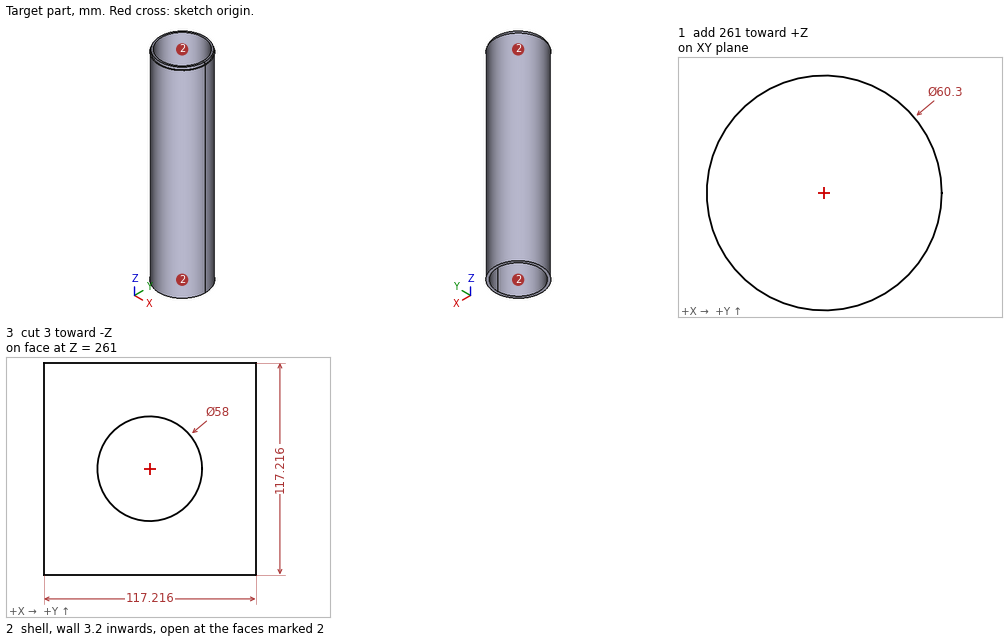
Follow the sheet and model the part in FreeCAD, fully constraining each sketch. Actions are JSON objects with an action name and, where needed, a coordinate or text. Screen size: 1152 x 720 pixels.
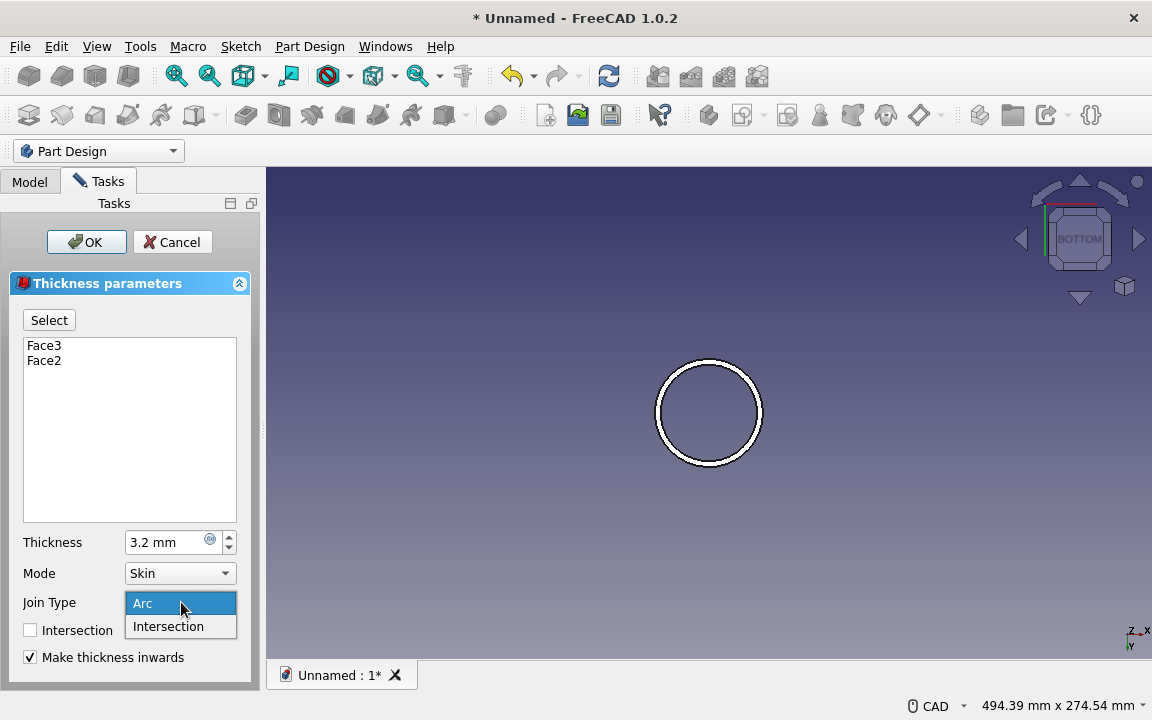
{"action": "left_click", "coordinate": [179, 626]}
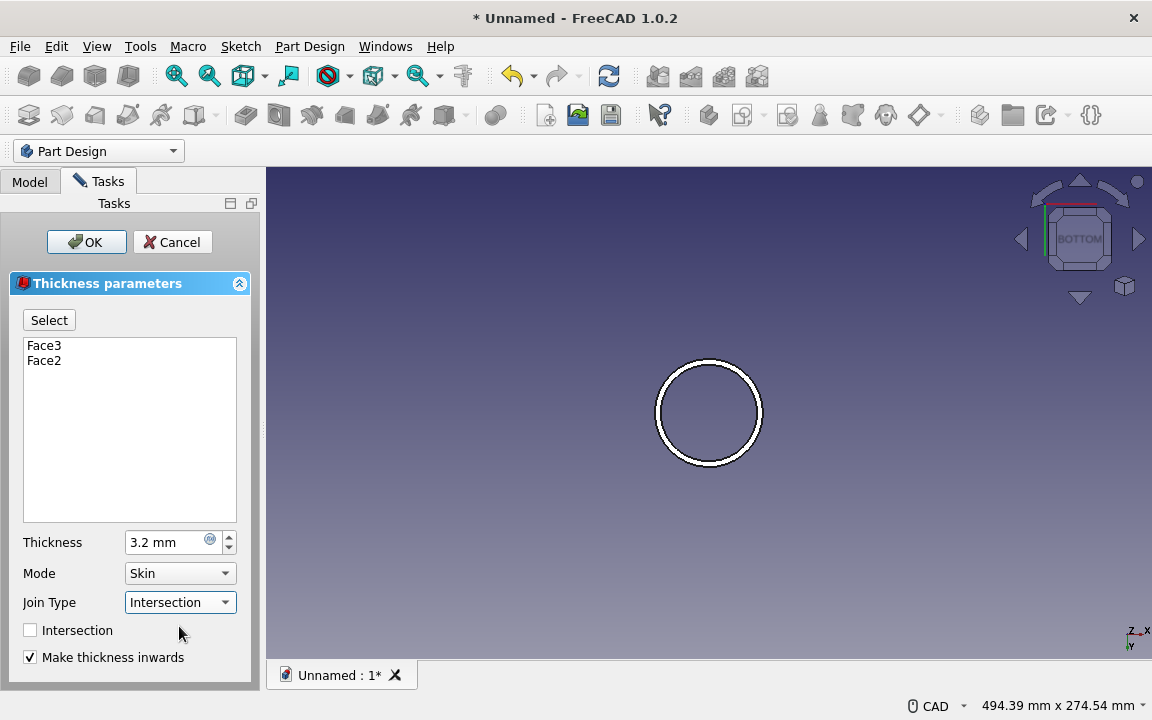
{"action": "left_click", "coordinate": [87, 242]}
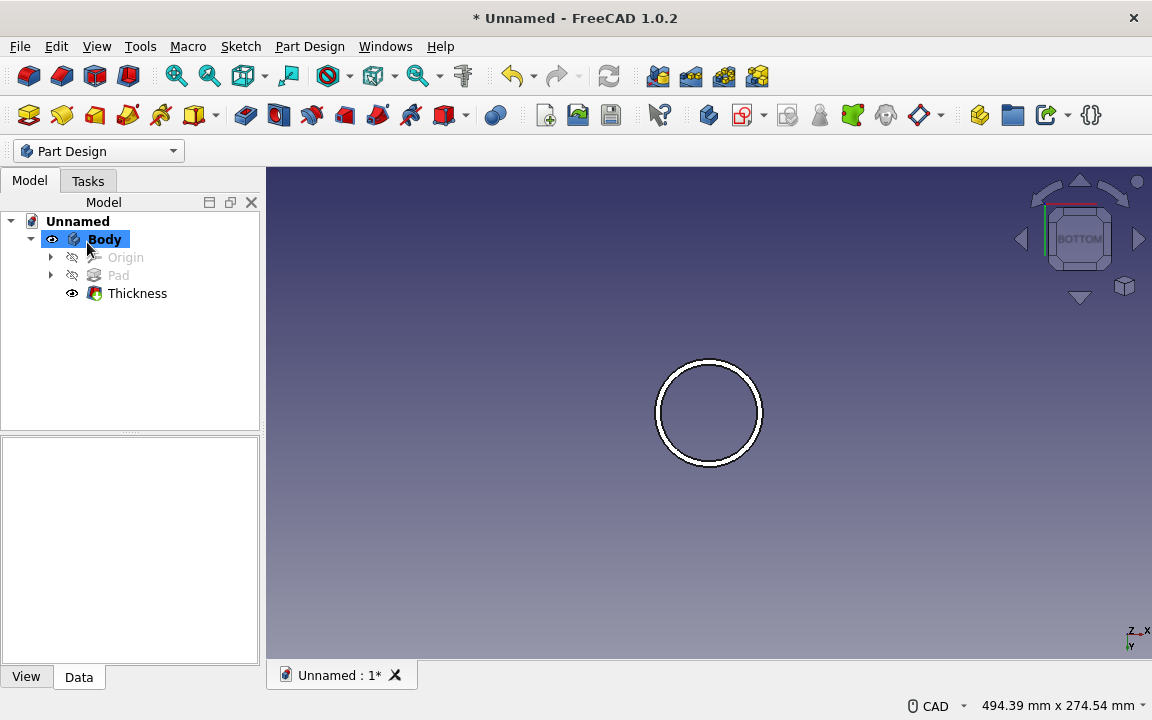
{"action": "key", "text": "v f"}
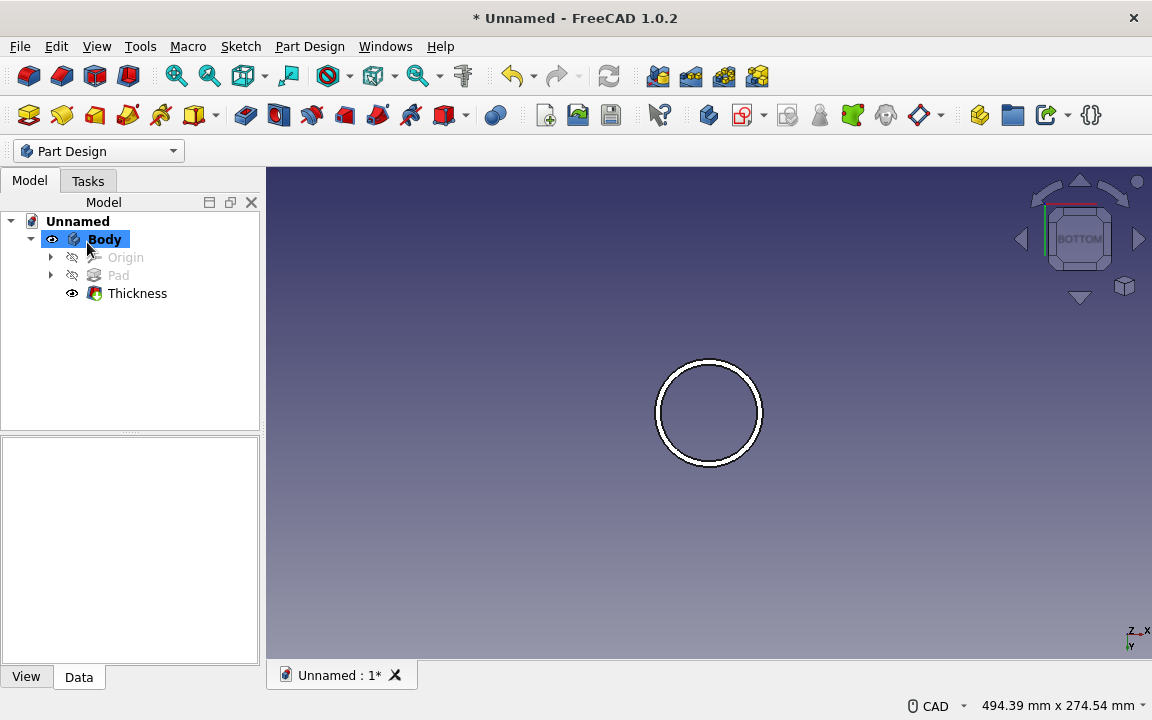
{"action": "key", "text": "0"}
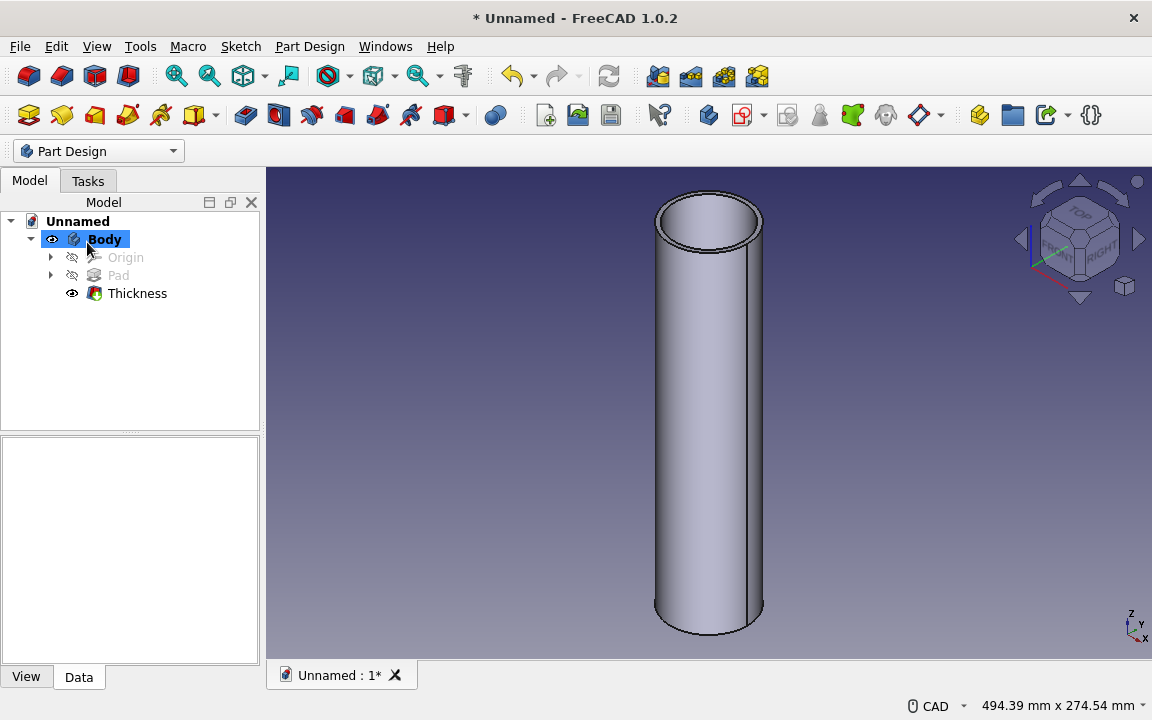
{"action": "scroll", "coordinate": [753, 208], "scroll_direction": "up", "scroll_amount": 15}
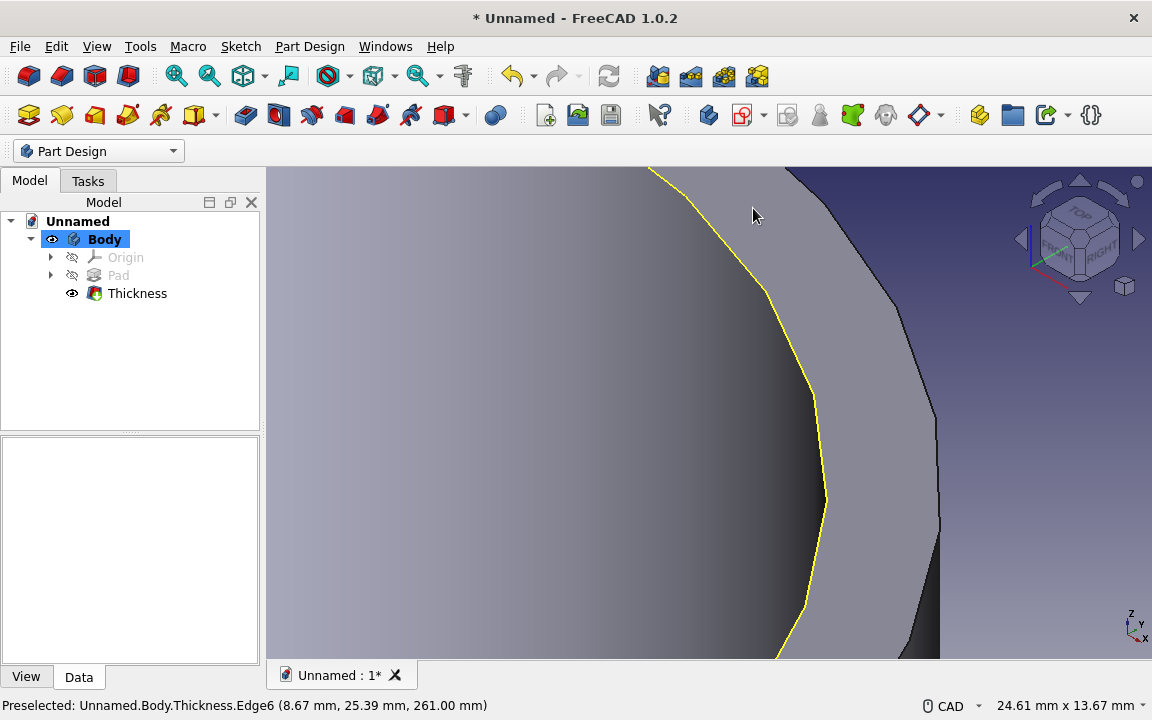
{"action": "left_click", "coordinate": [734, 233]}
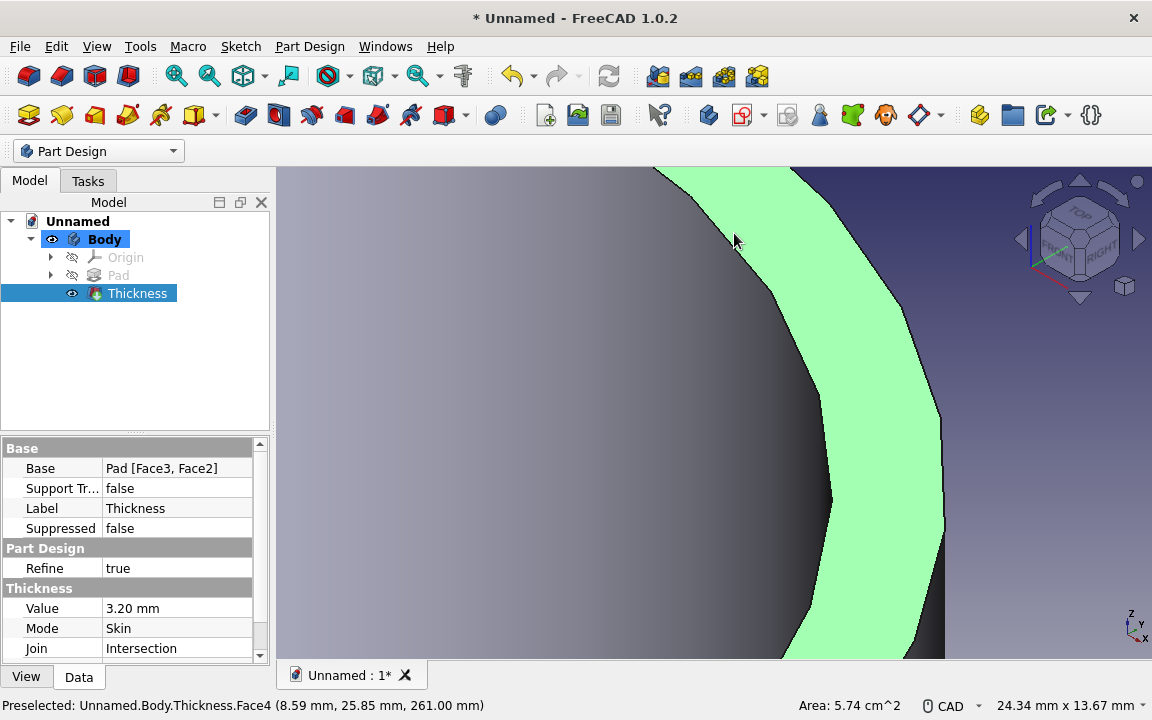
{"action": "left_click", "coordinate": [742, 116]}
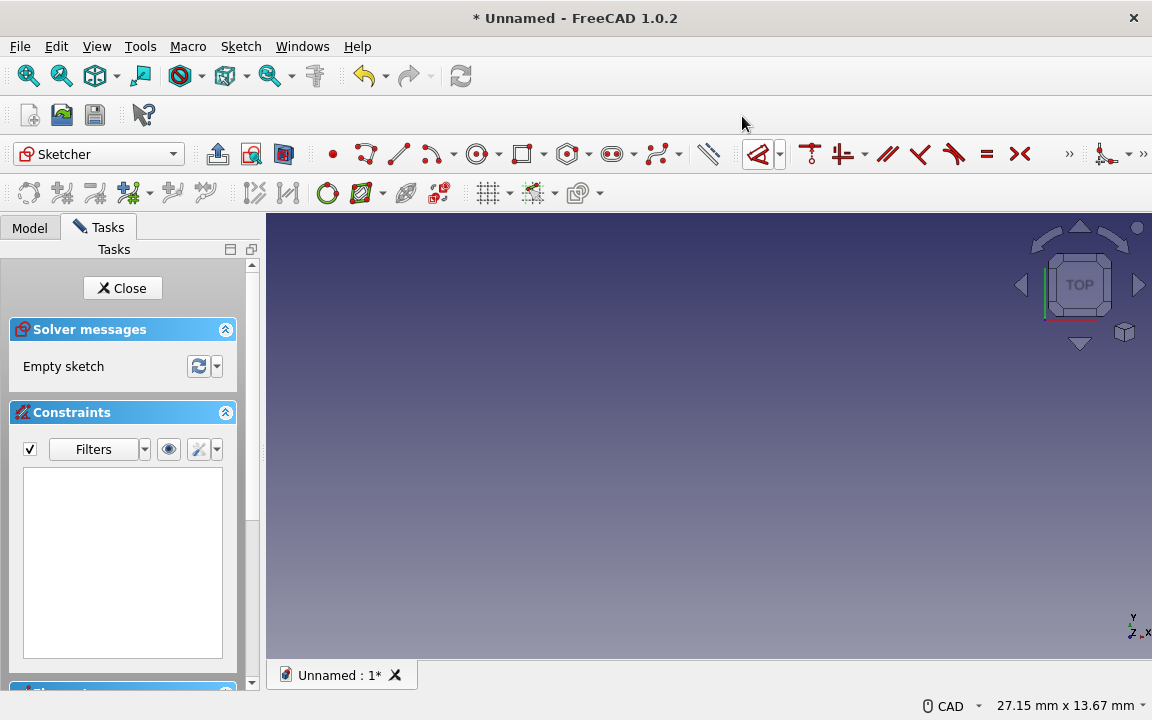
{"action": "scroll", "coordinate": [563, 276], "scroll_direction": "down", "scroll_amount": 13}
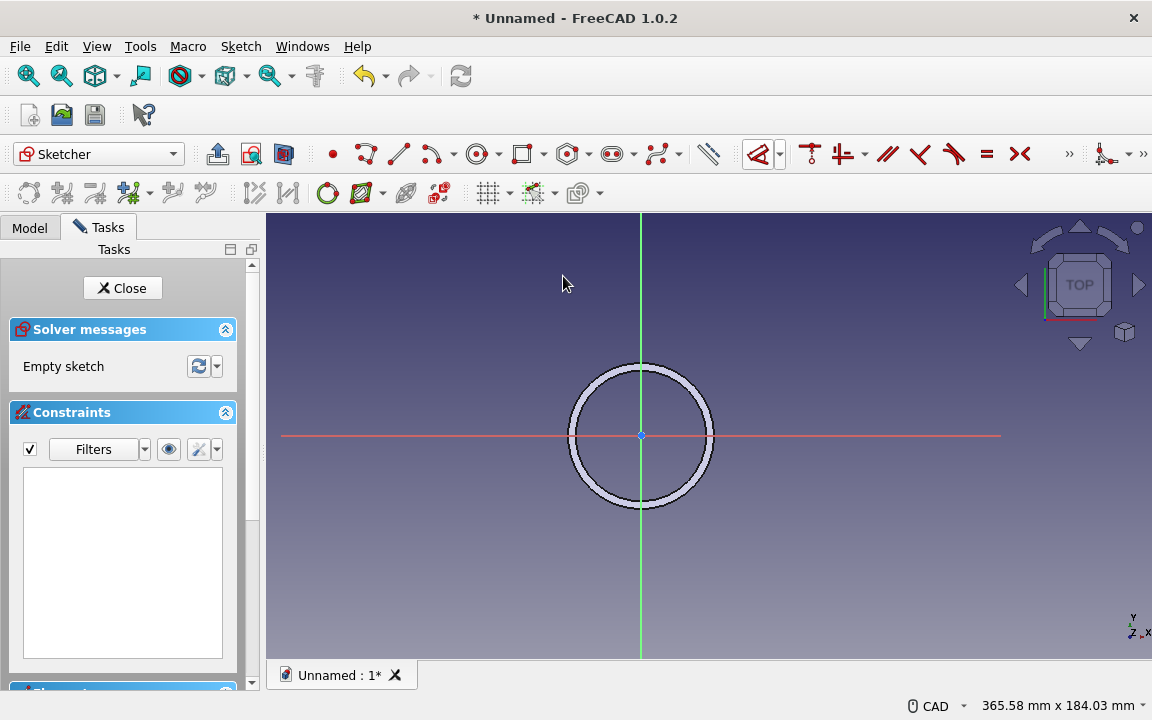
{"action": "key", "text": "g v"}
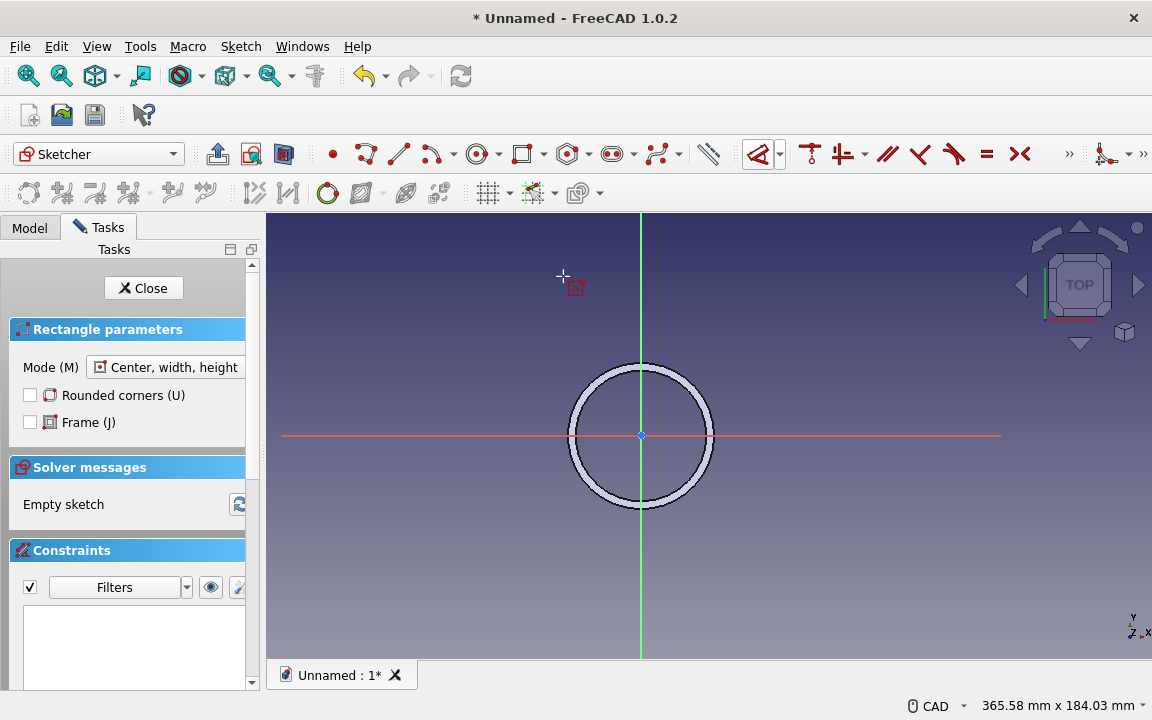
{"action": "left_click", "coordinate": [641, 436]}
{"action": "mouse_move", "coordinate": [783, 294]}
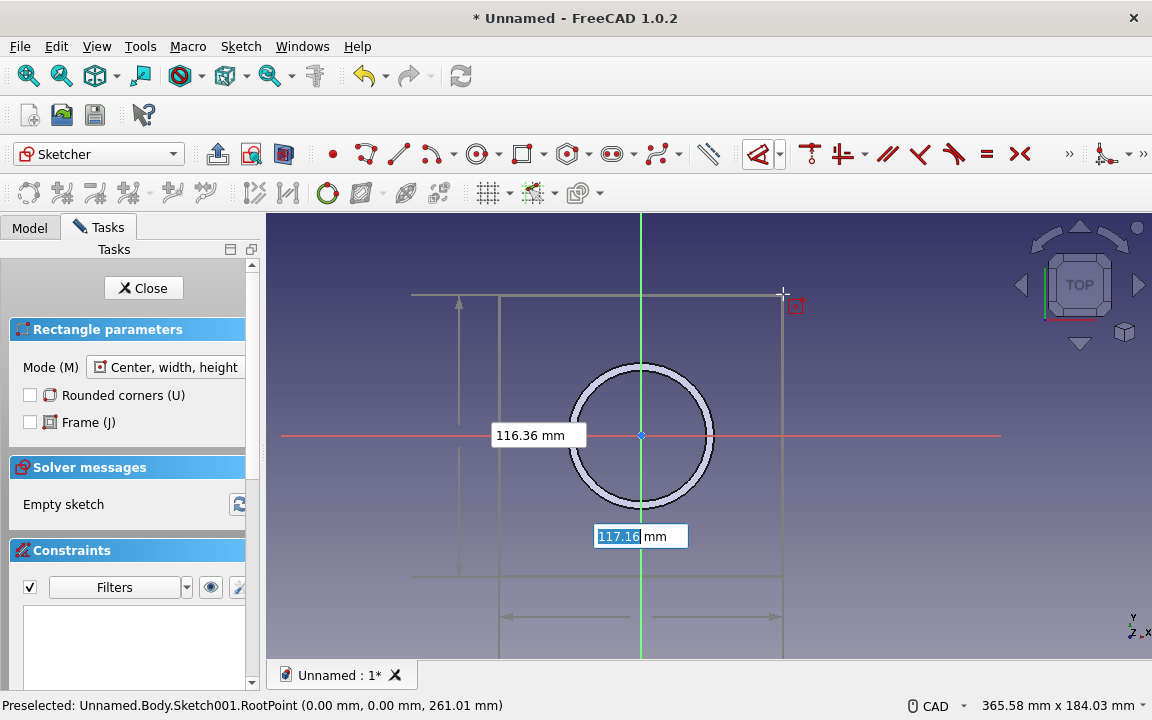
{"action": "type", "text": "117.216"}
{"action": "key", "text": "Tab"}
{"action": "type", "text": "117.216"}
{"action": "key", "text": "Return"}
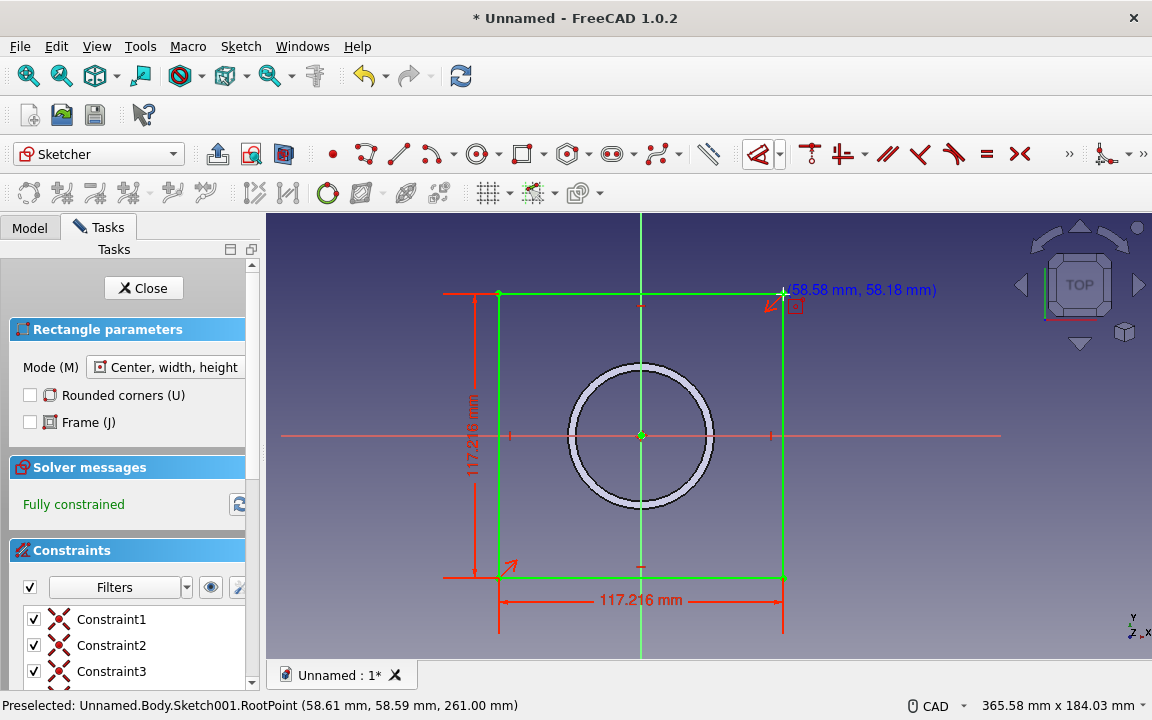
{"action": "key", "text": "g c"}